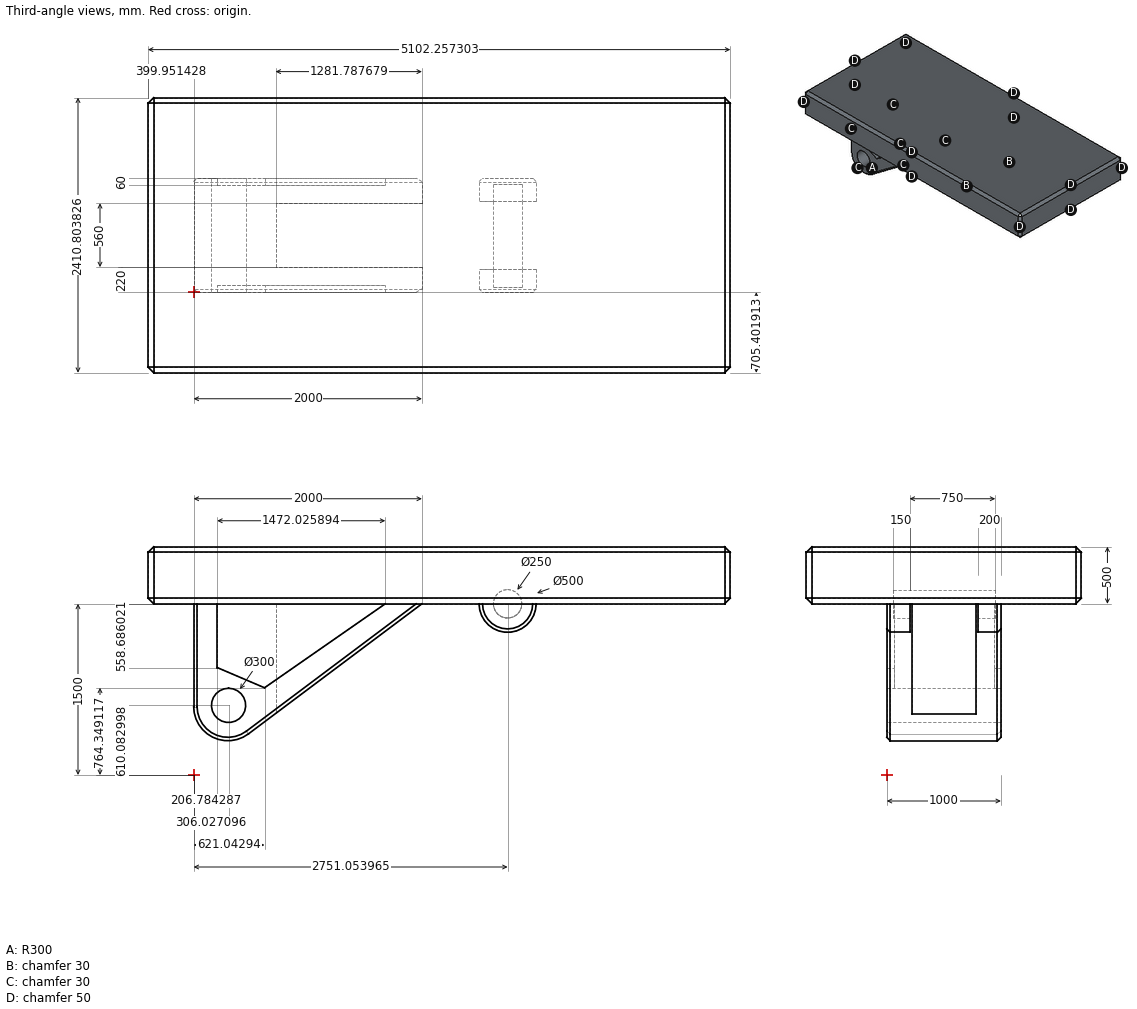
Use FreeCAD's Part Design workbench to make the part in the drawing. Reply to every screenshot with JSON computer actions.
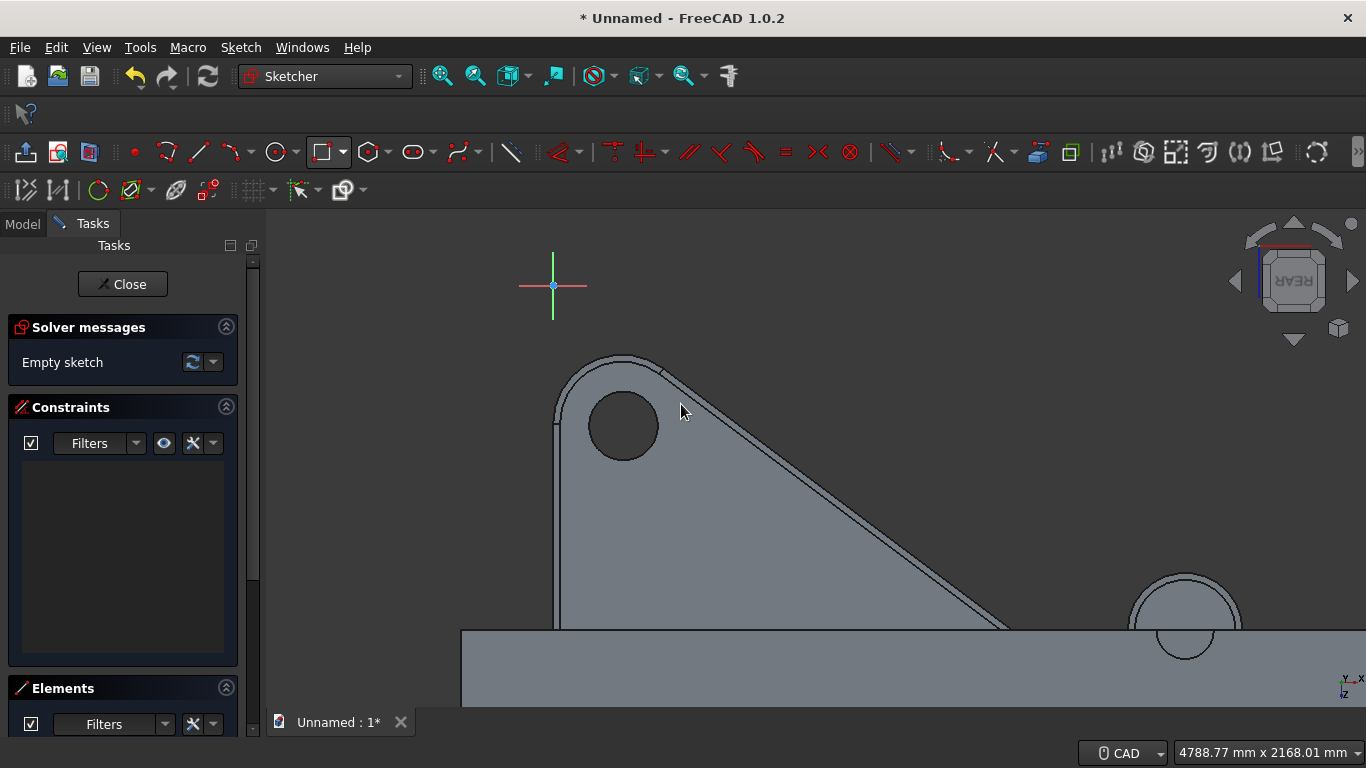
{"action": "left_click", "coordinate": [168, 152]}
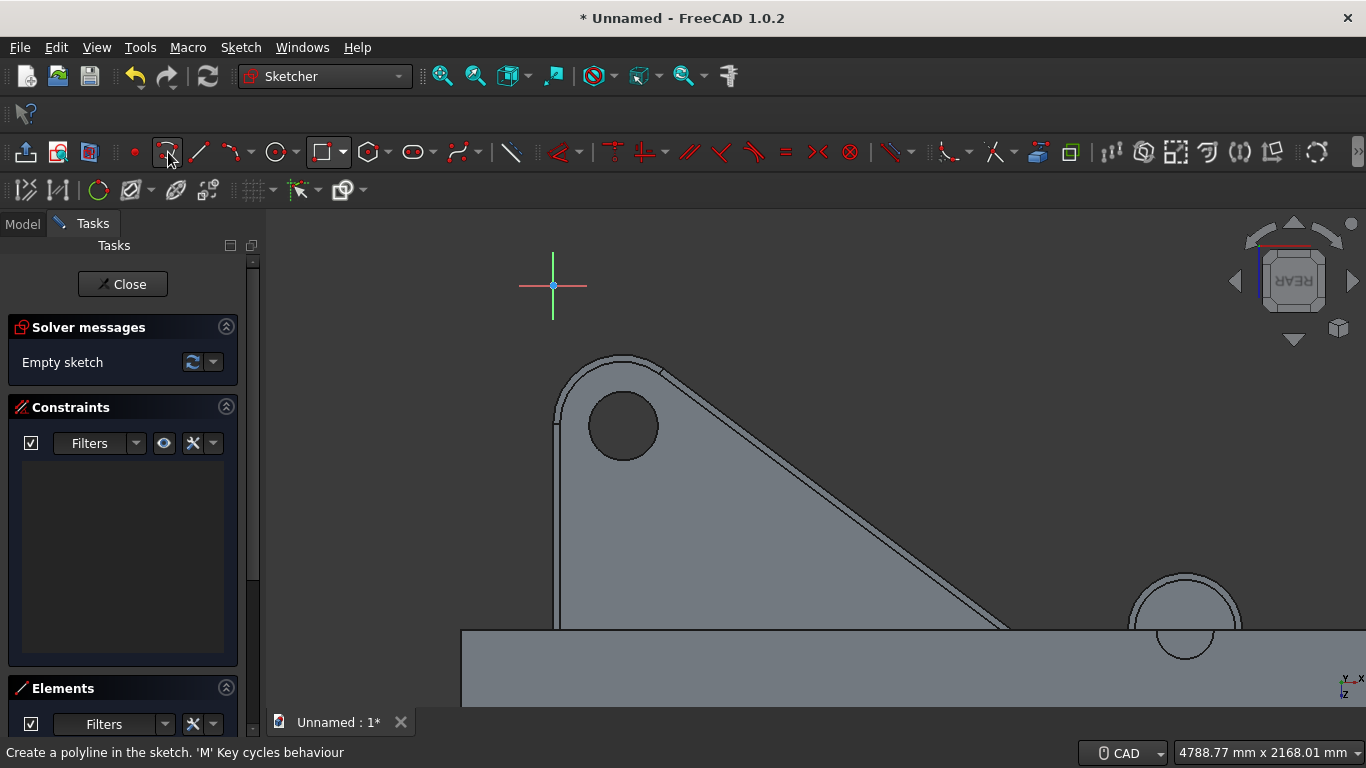
{"action": "left_click", "coordinate": [601, 502]}
{"action": "left_click", "coordinate": [601, 630]}
{"action": "left_click", "coordinate": [939, 630]}
{"action": "left_click", "coordinate": [696, 461]}
{"action": "left_click", "coordinate": [601, 503]}
{"action": "key", "text": "Escape"}
{"action": "key", "text": "Escape"}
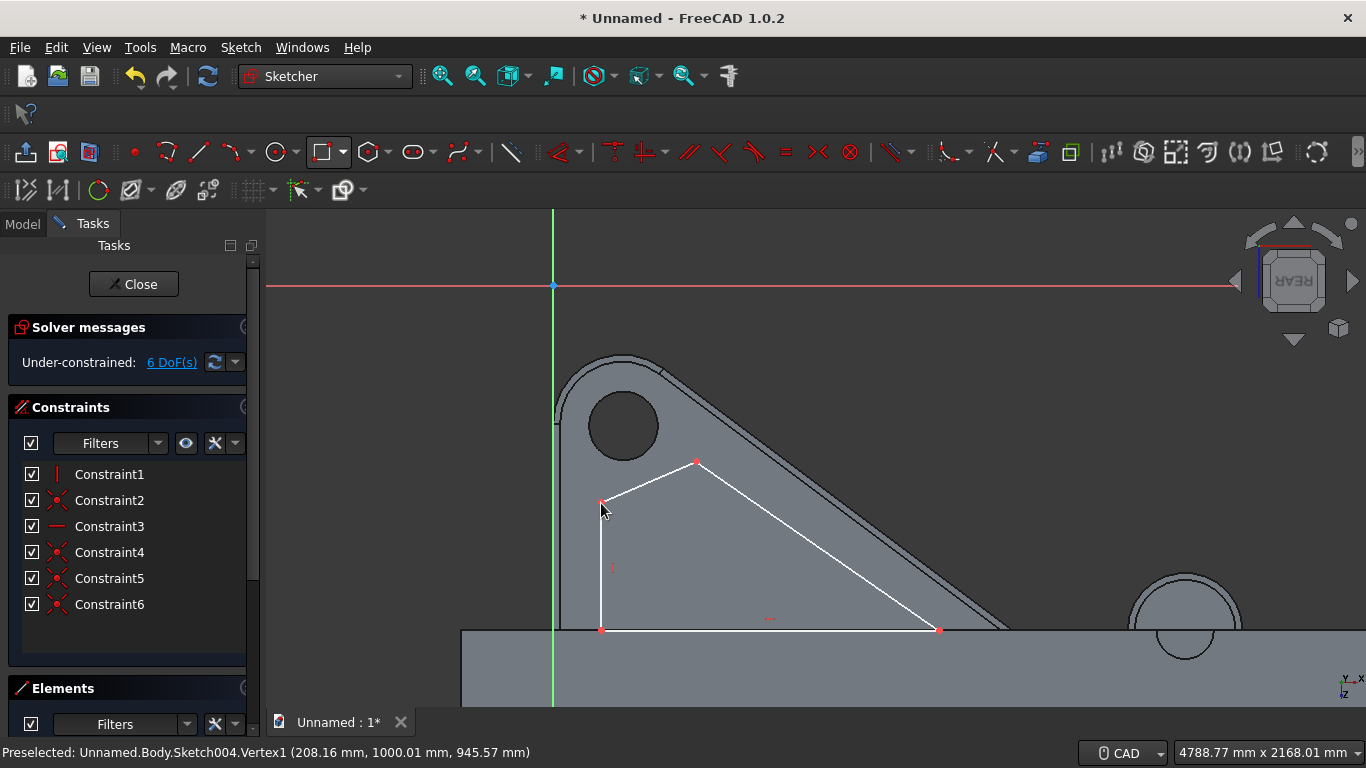
{"action": "key", "text": "d"}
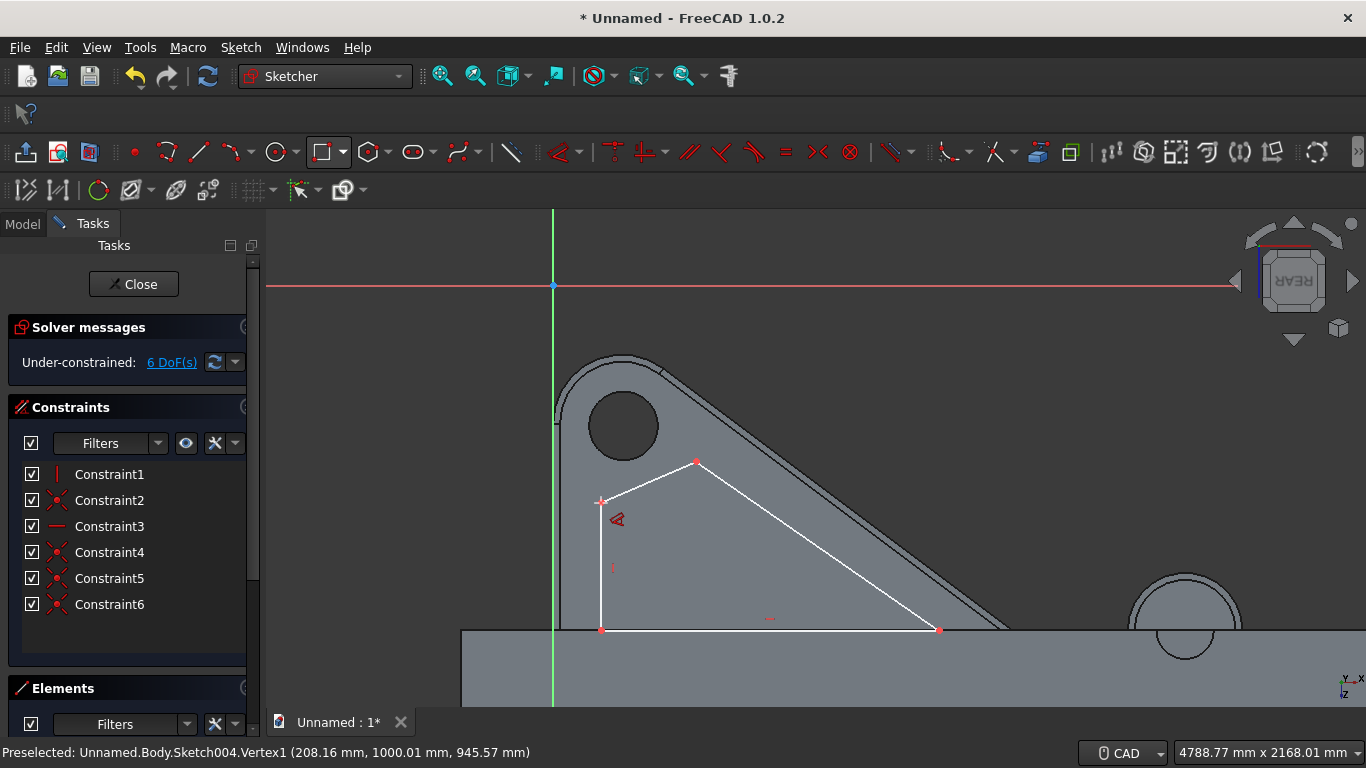
{"action": "left_click", "coordinate": [601, 631]}
{"action": "left_click", "coordinate": [519, 458]}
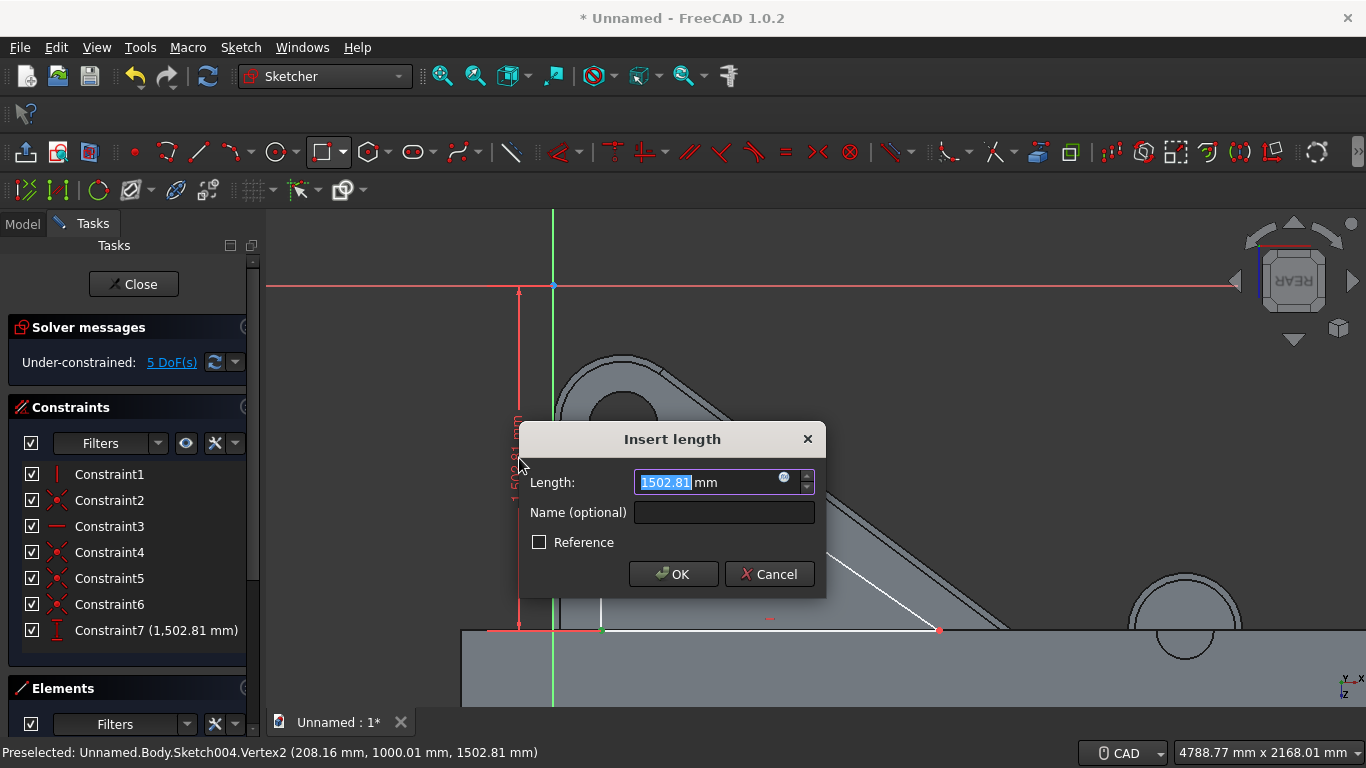
{"action": "type", "text": "1500"}
{"action": "key", "text": "Return"}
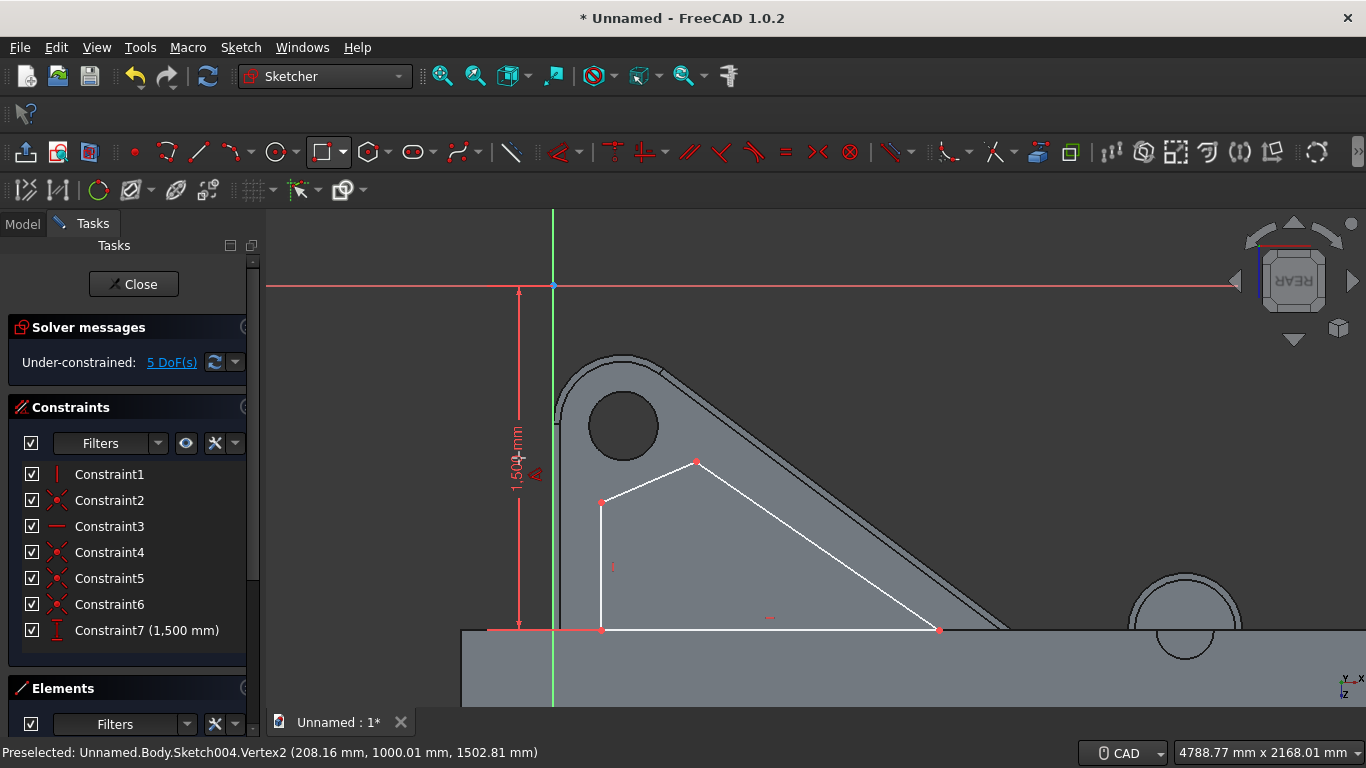
{"action": "left_click", "coordinate": [601, 541]}
{"action": "left_click", "coordinate": [567, 567]}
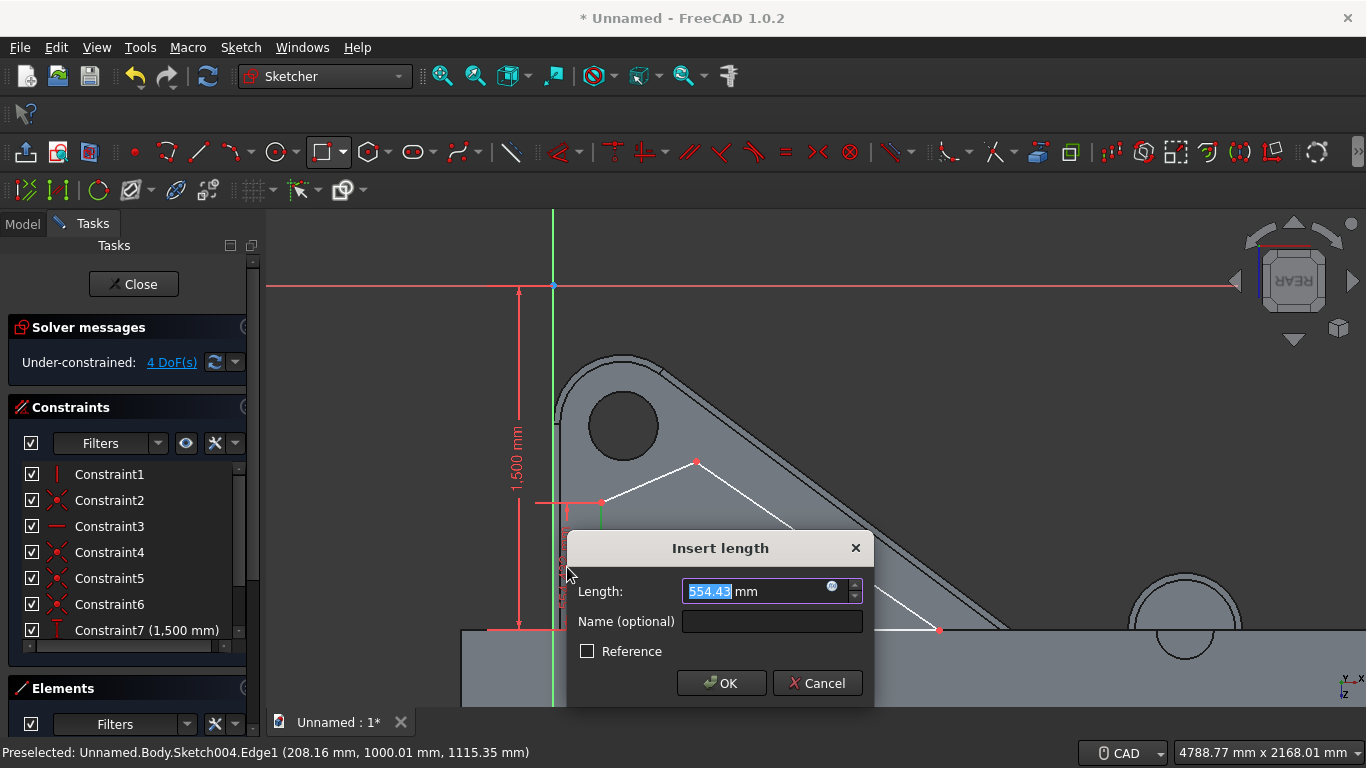
{"action": "type", "text": "558.686021"}
{"action": "key", "text": "Return"}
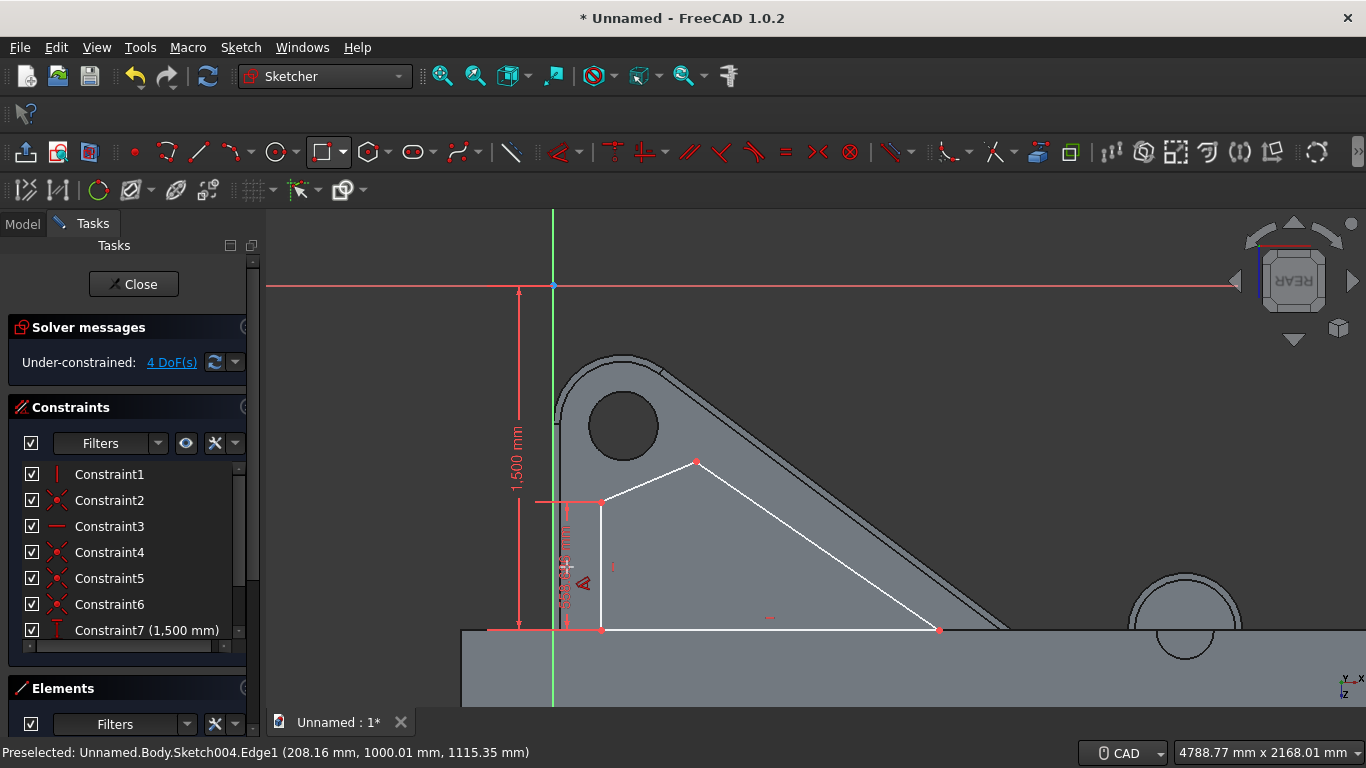
{"action": "left_click", "coordinate": [696, 462]}
{"action": "left_click", "coordinate": [625, 252]}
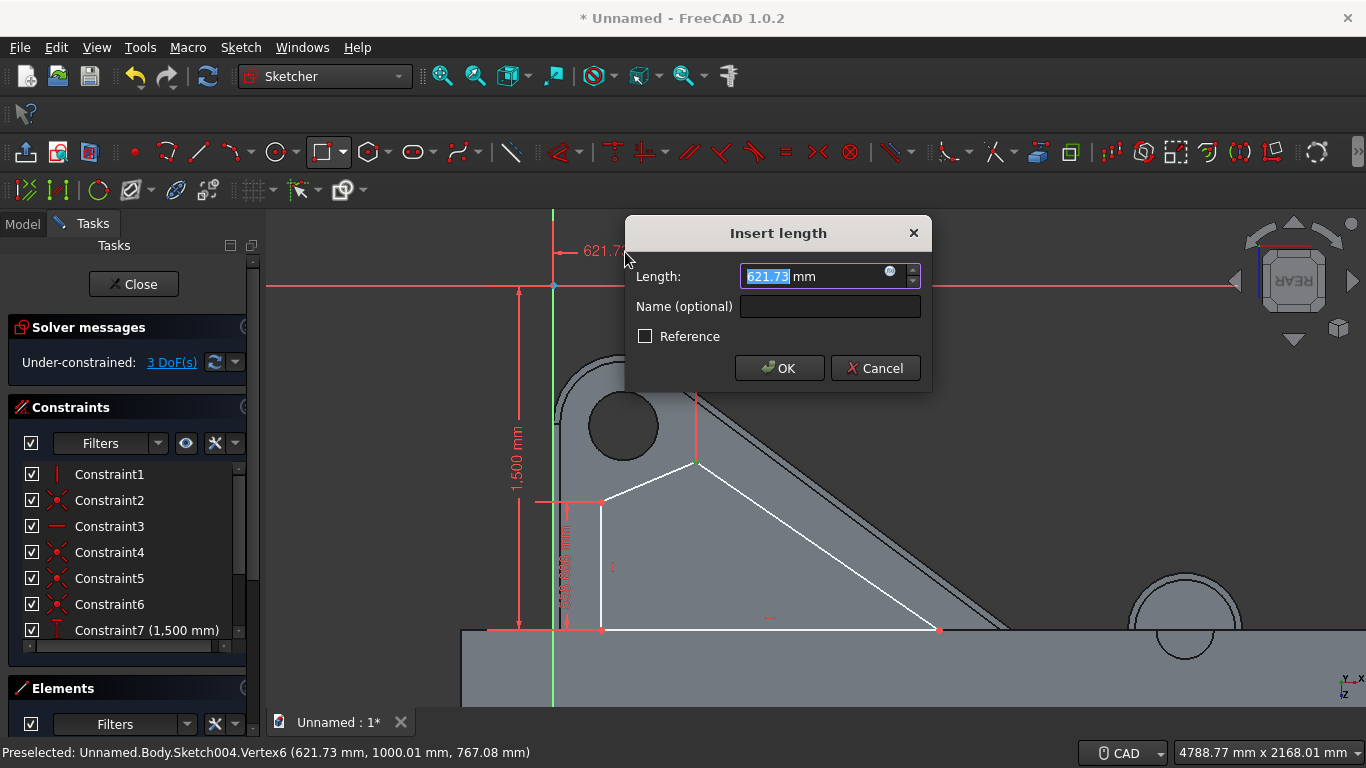
{"action": "type", "text": "621.04294"}
{"action": "key", "text": "Return"}